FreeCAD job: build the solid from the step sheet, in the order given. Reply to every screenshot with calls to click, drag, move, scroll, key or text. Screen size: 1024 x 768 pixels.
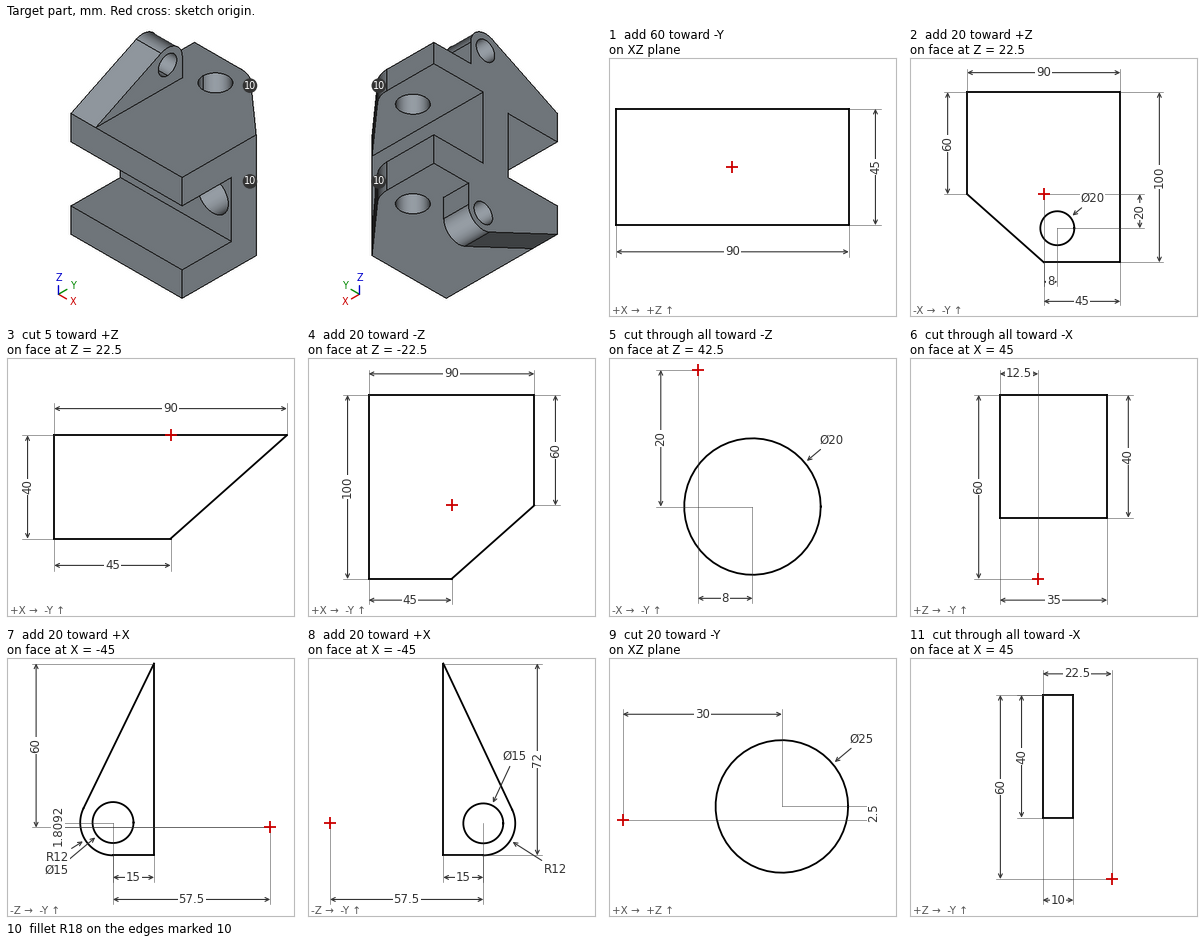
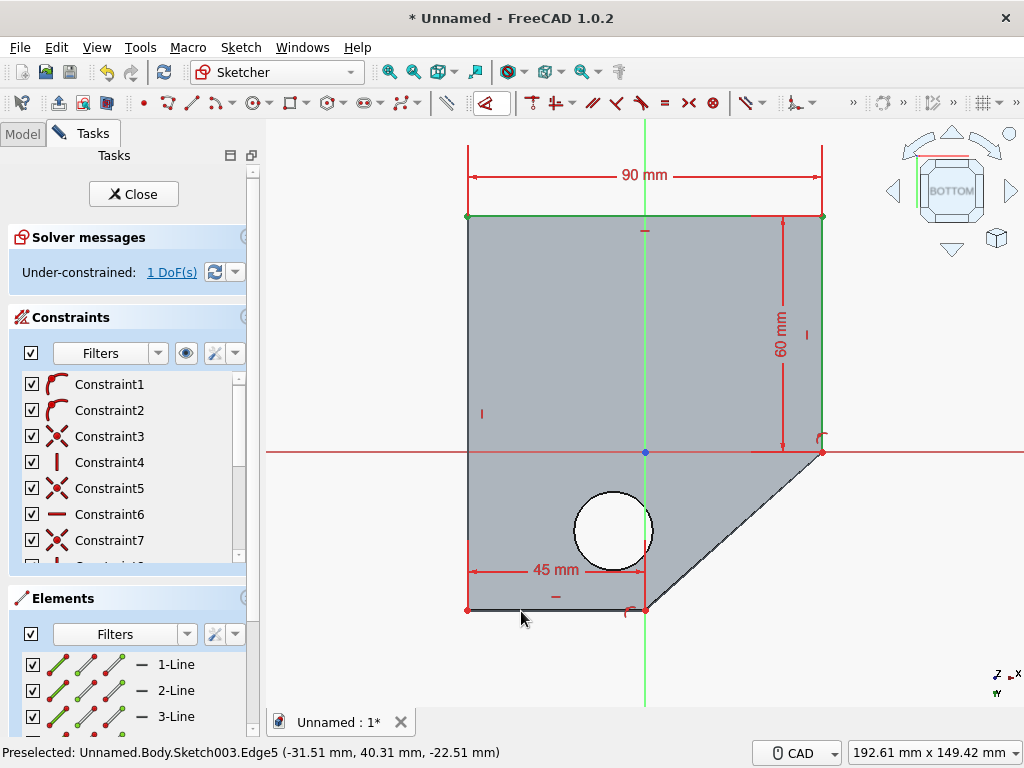
click(468, 335)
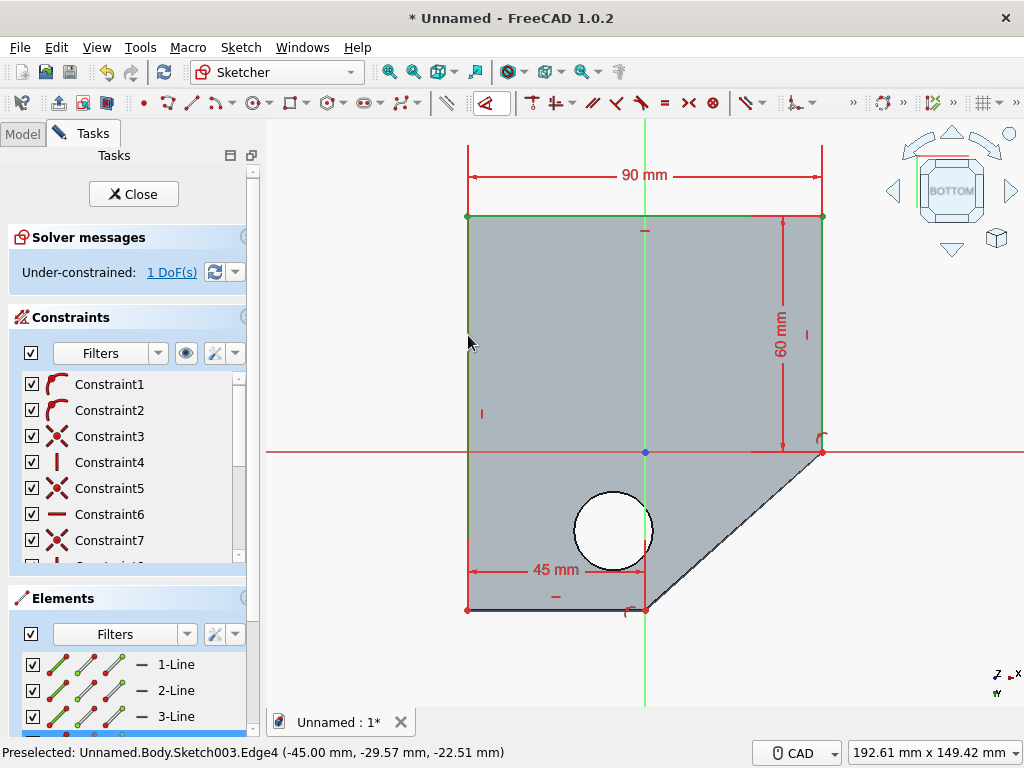
key(i)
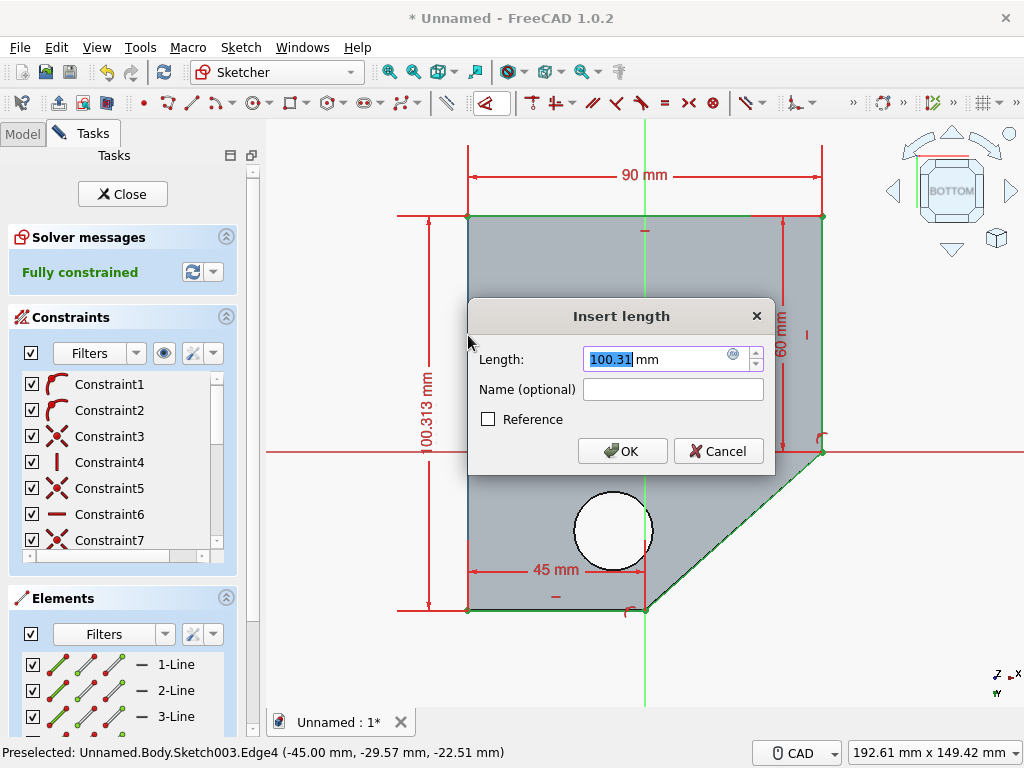
text(100)
key(Return)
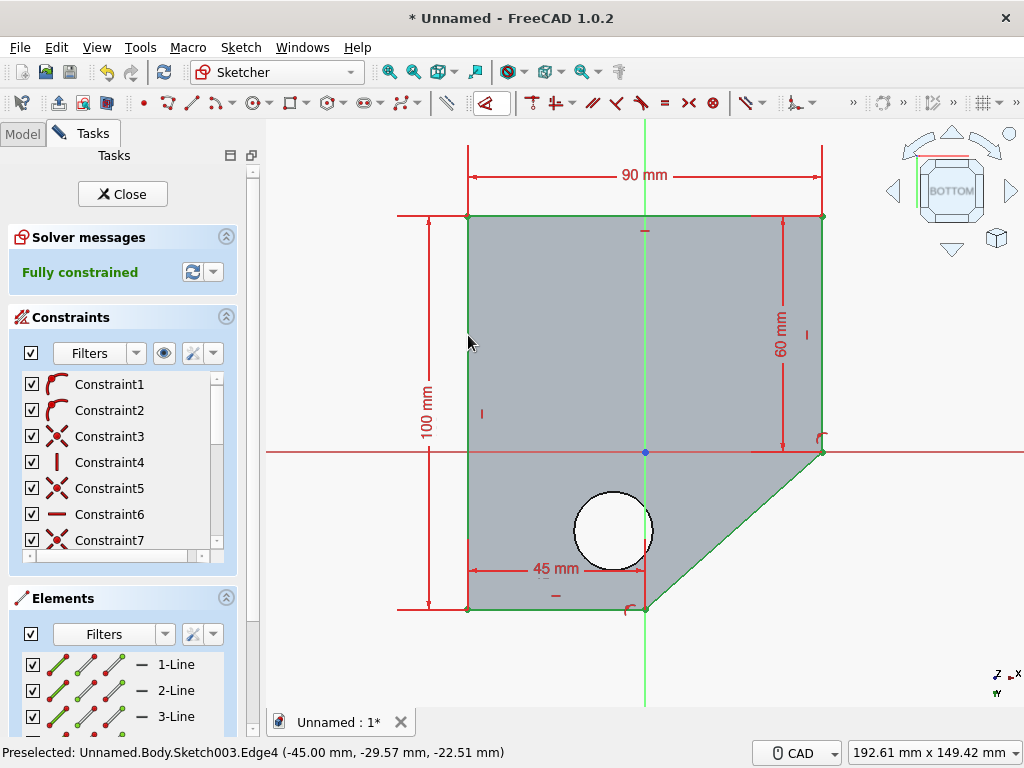
click(123, 194)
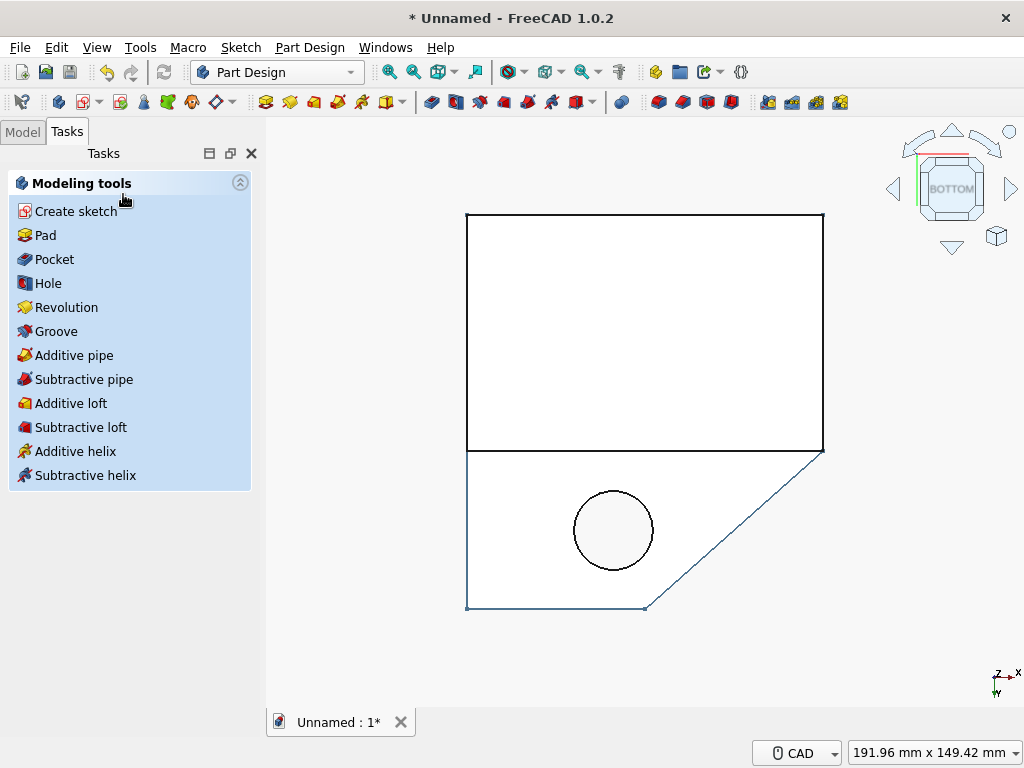
click(266, 102)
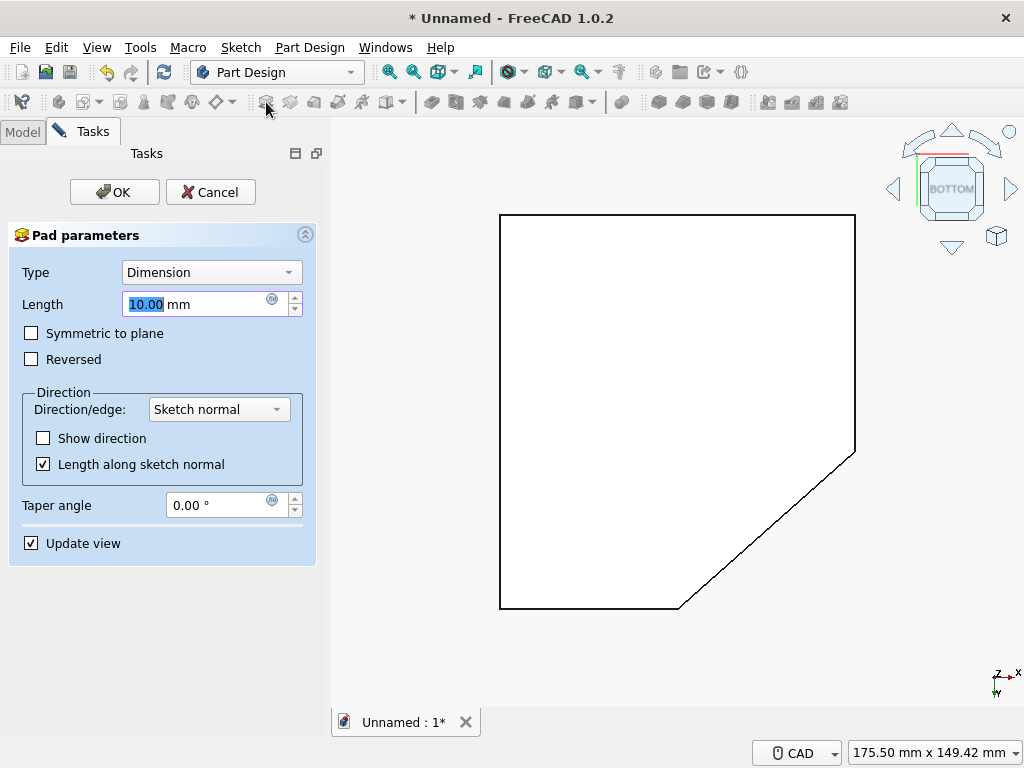
text(20)
key(Tab)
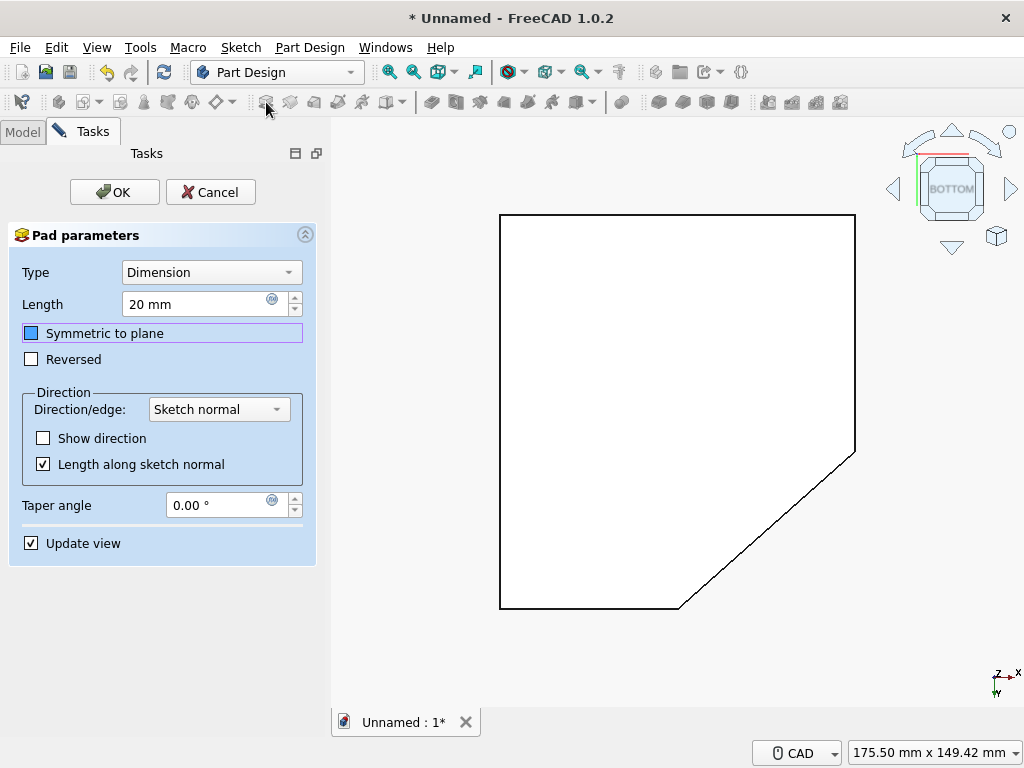
click(115, 192)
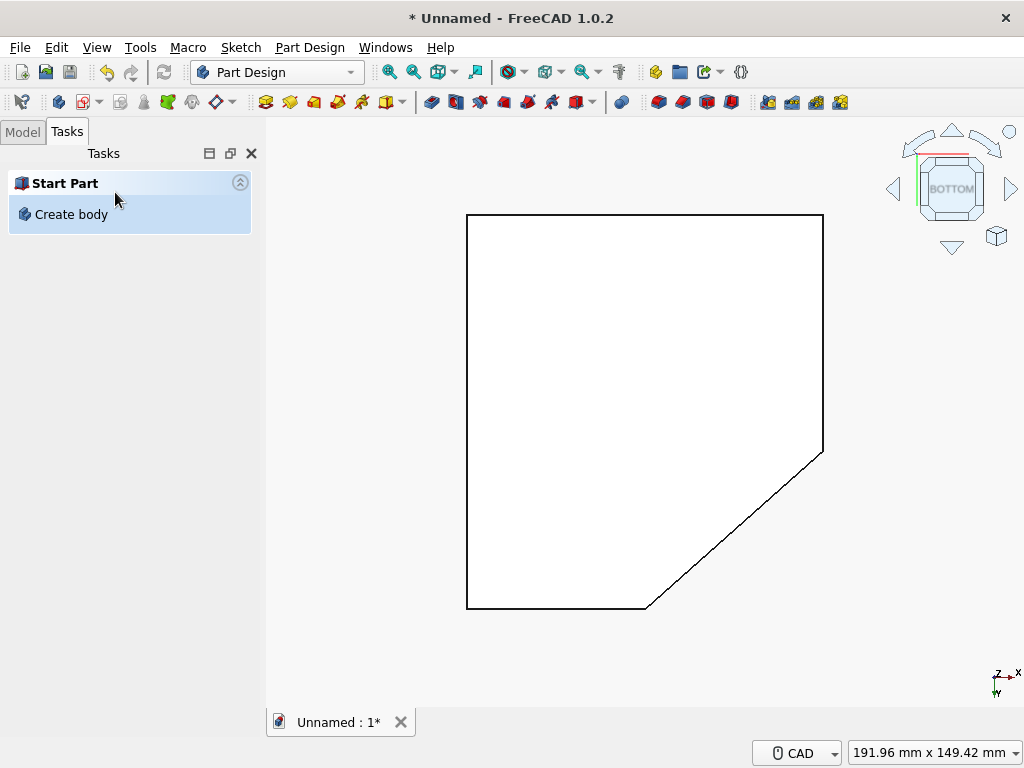
key(0)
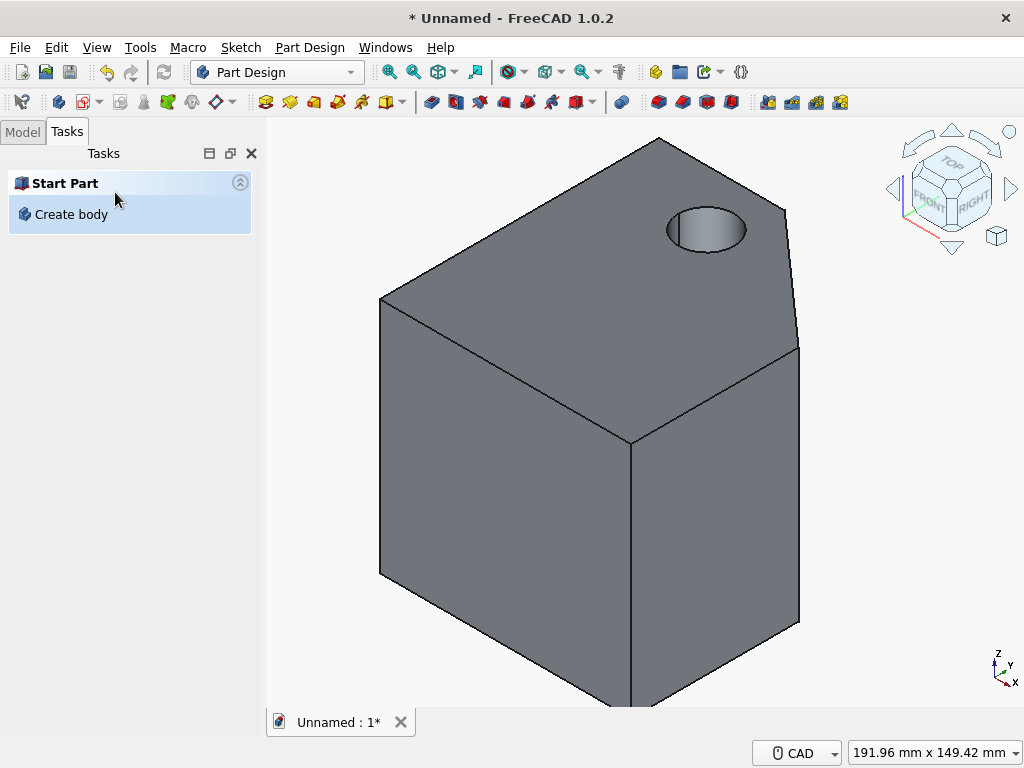
click(390, 72)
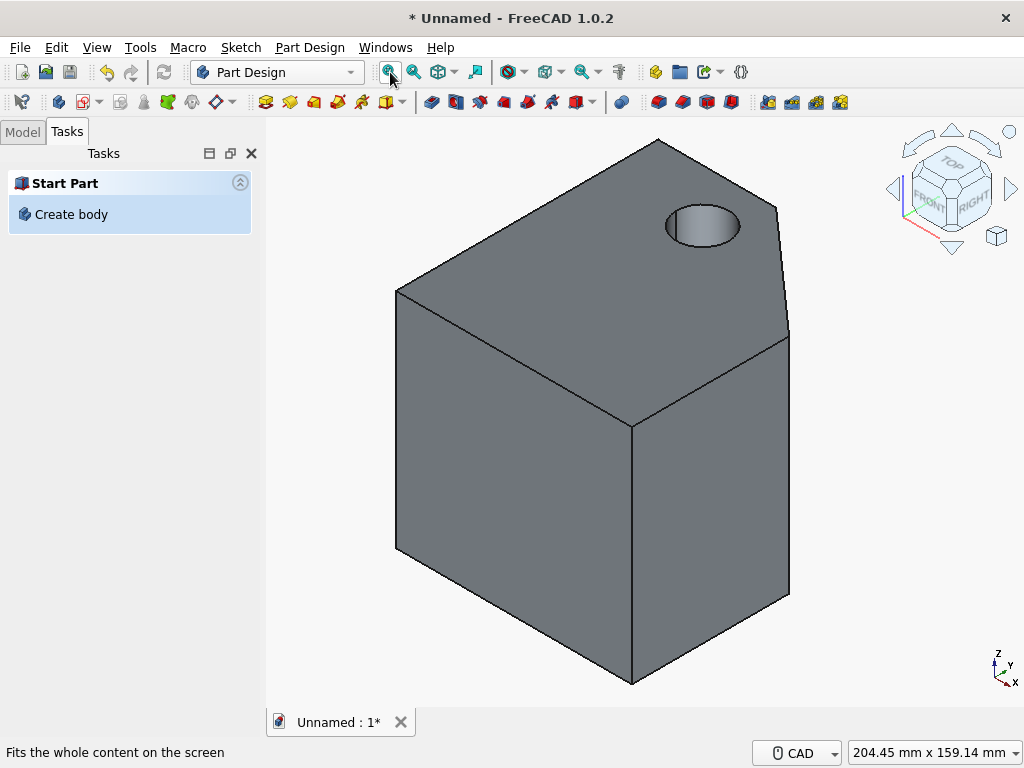
click(608, 304)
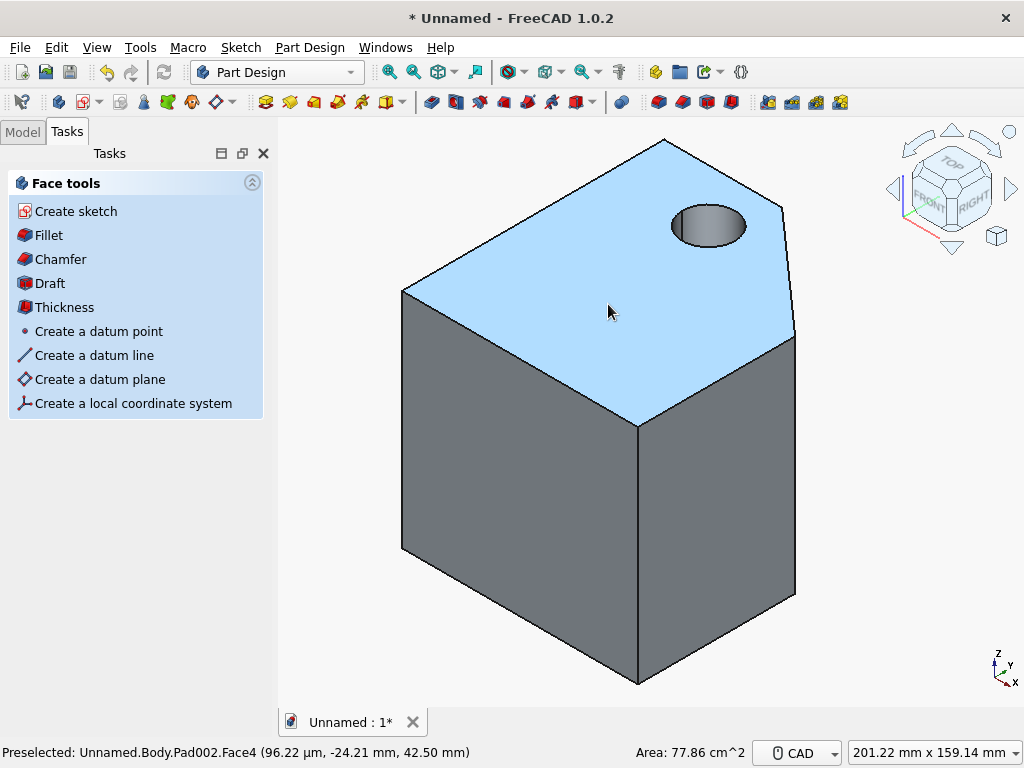
click(84, 102)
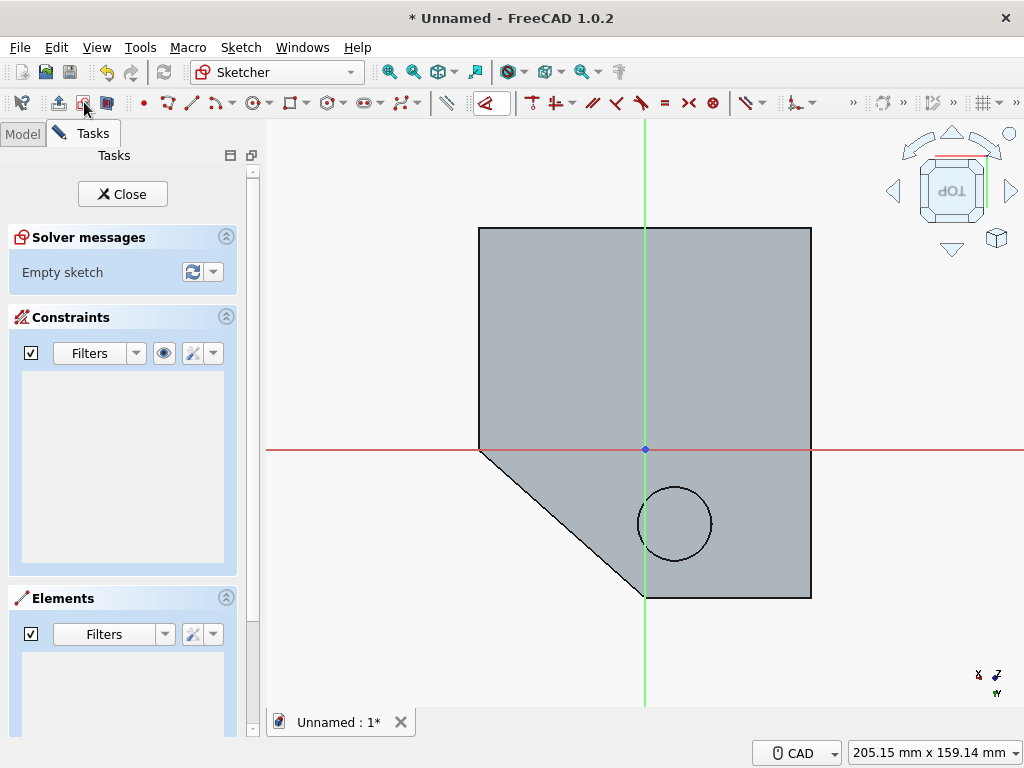
scroll(717, 545, up, 6)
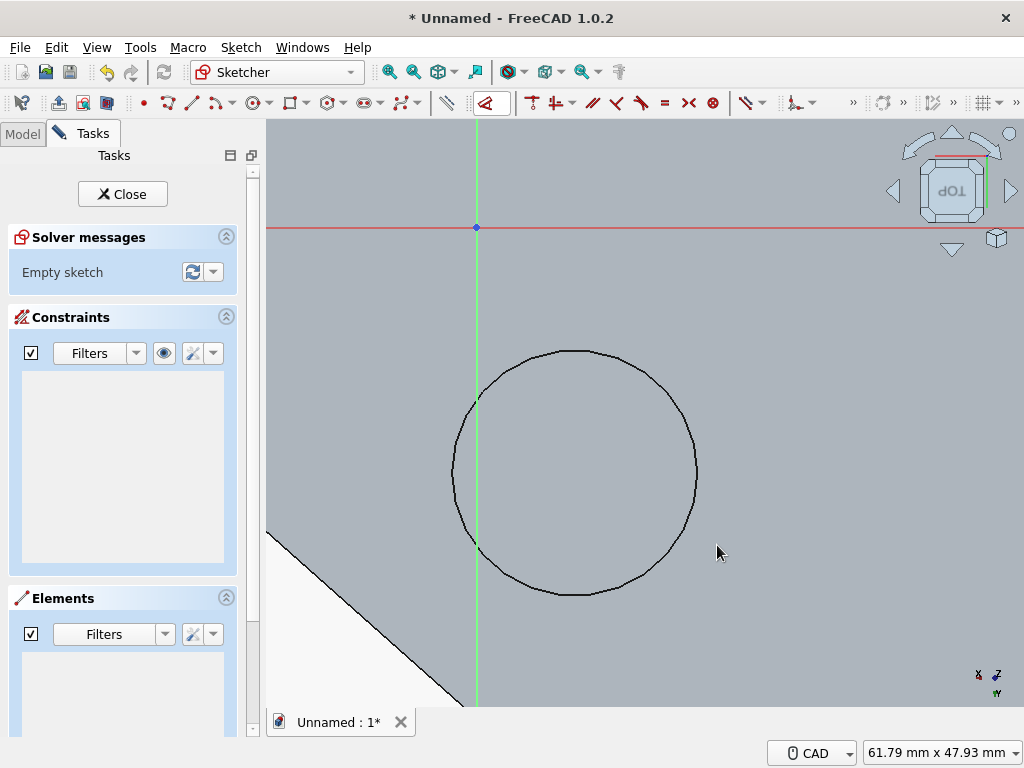
key(g)
key(c)